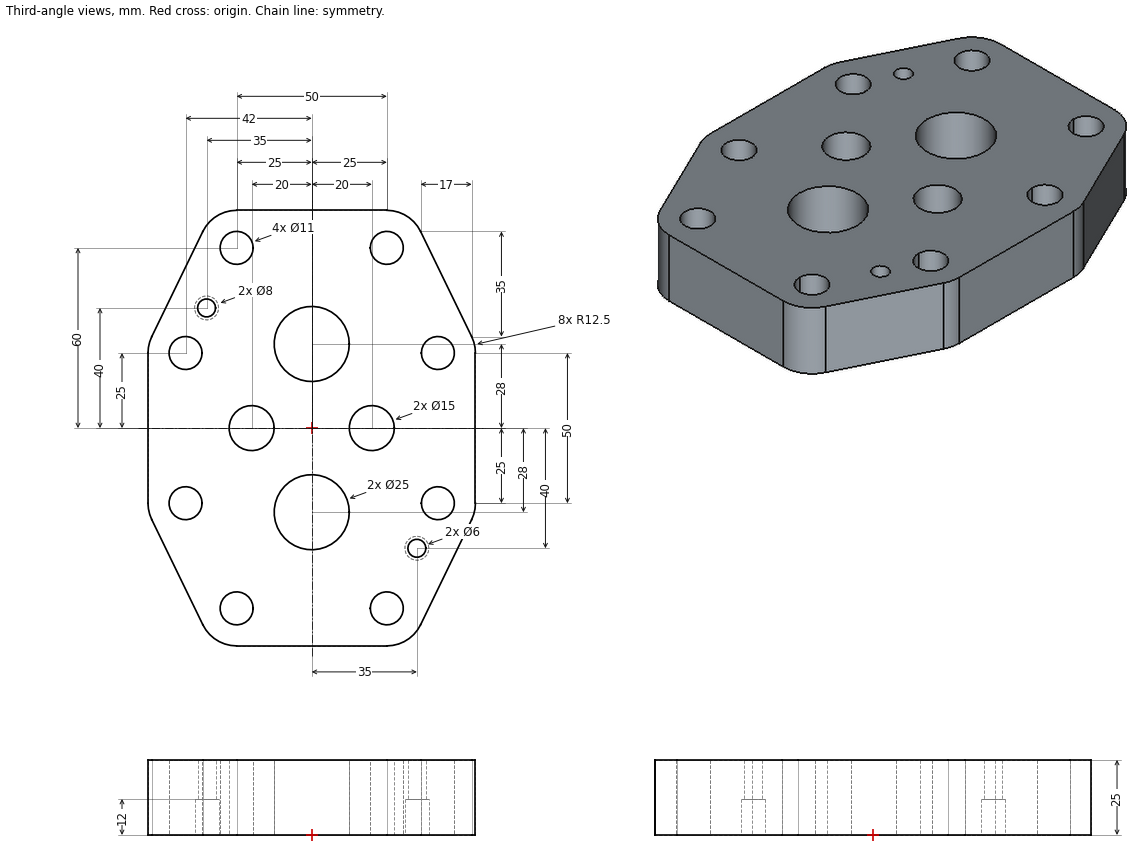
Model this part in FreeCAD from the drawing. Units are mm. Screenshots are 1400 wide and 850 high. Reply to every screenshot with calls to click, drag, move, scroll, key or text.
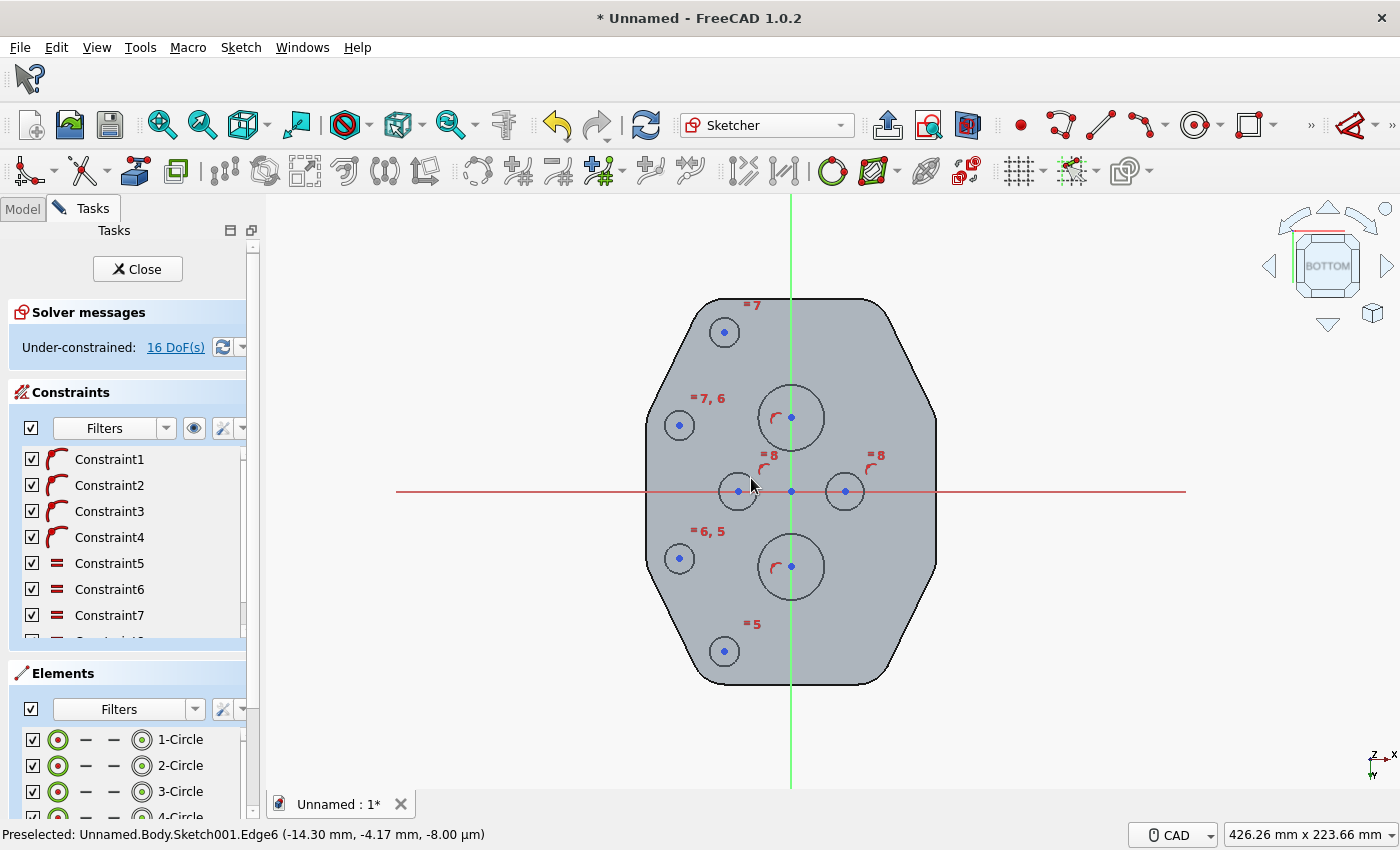
click(815, 395)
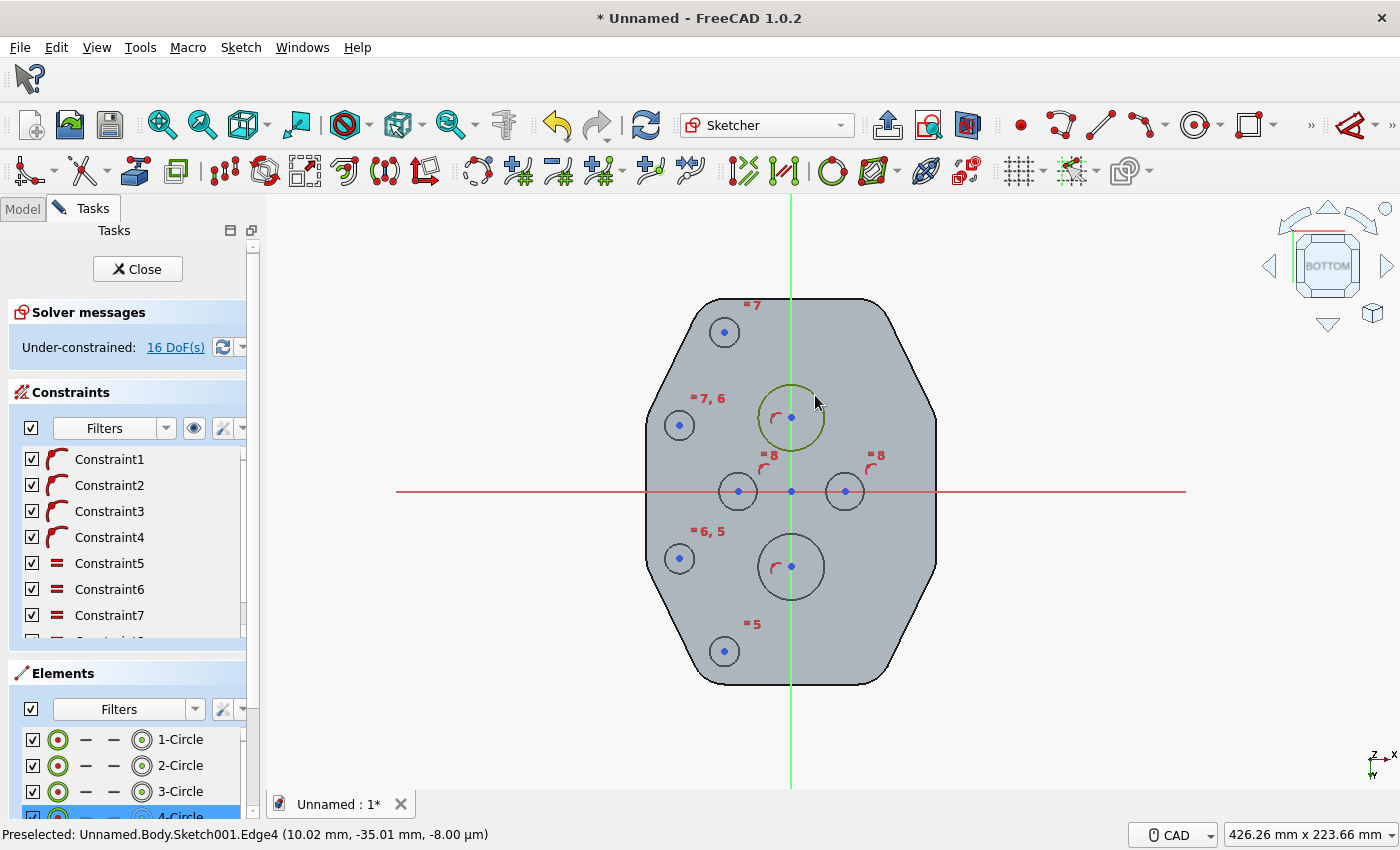
click(815, 544)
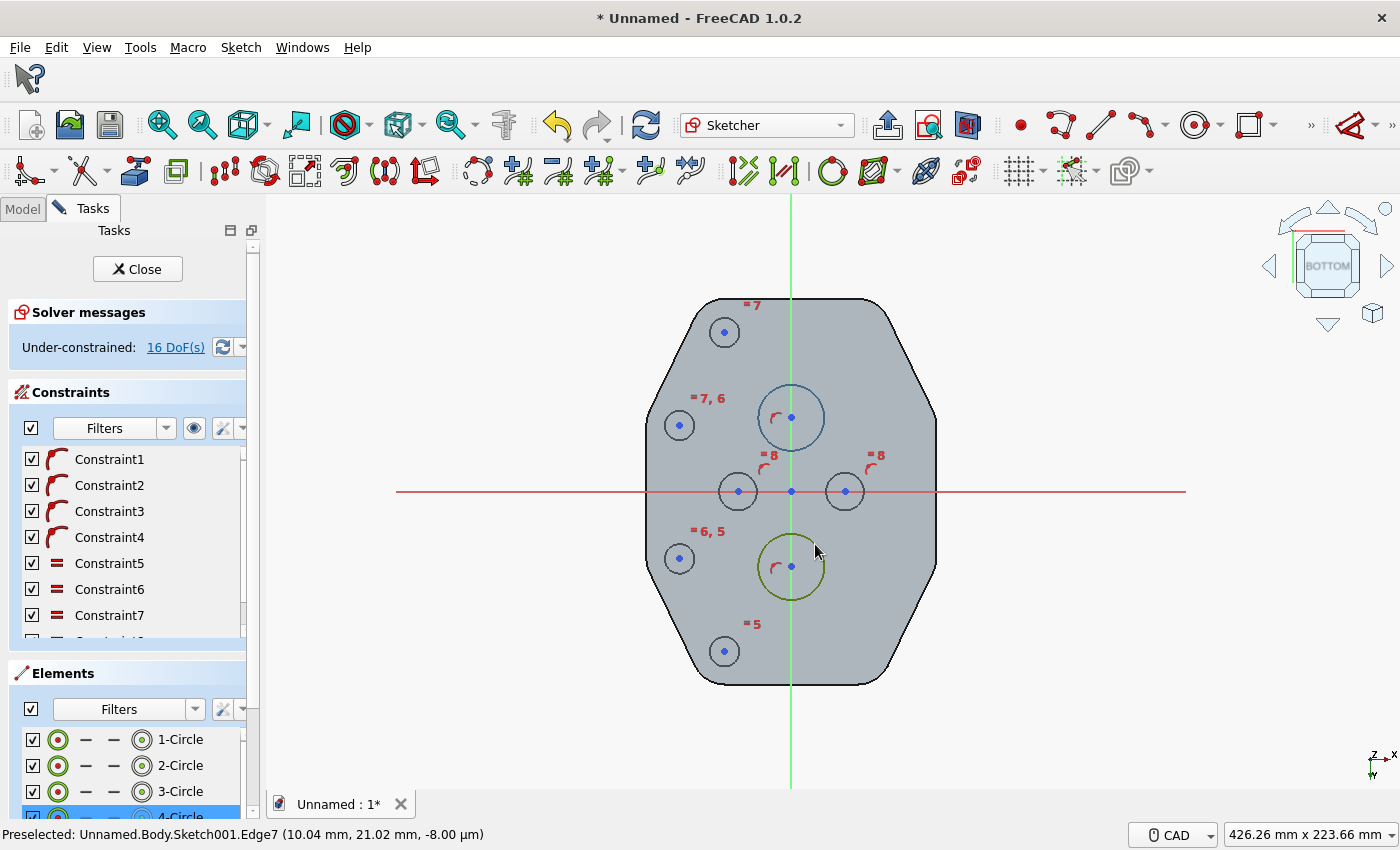
key(e)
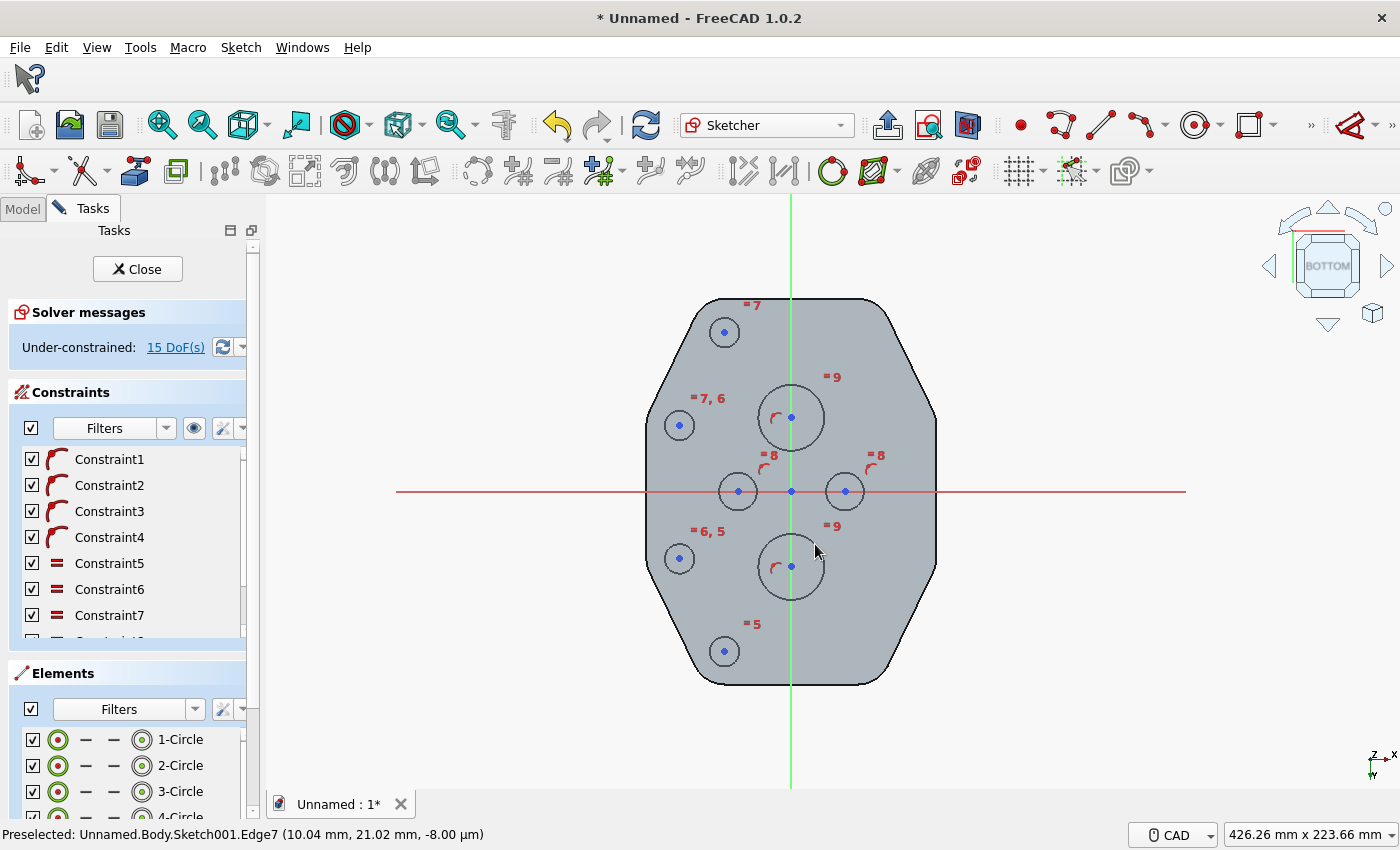
click(680, 559)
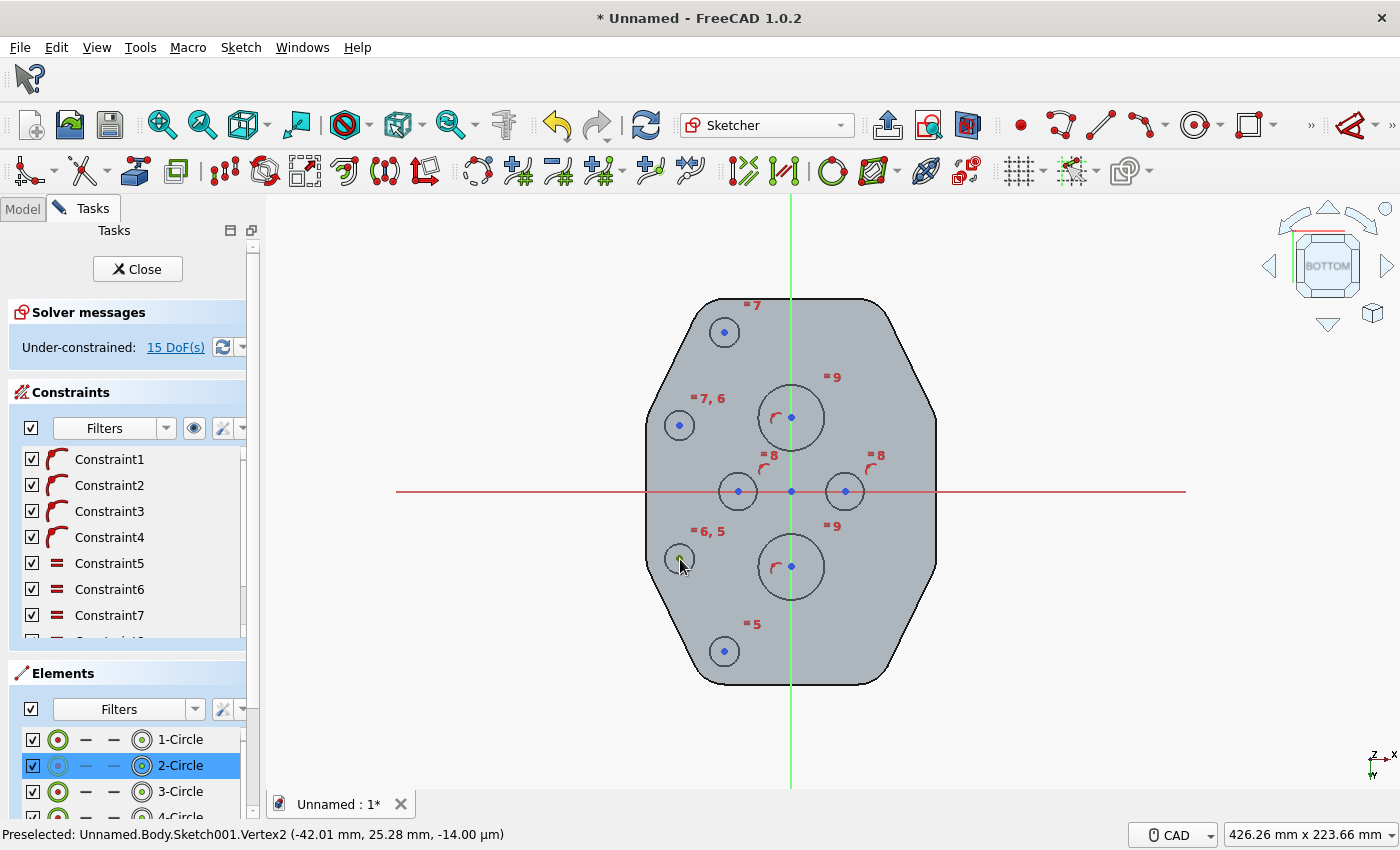
click(680, 426)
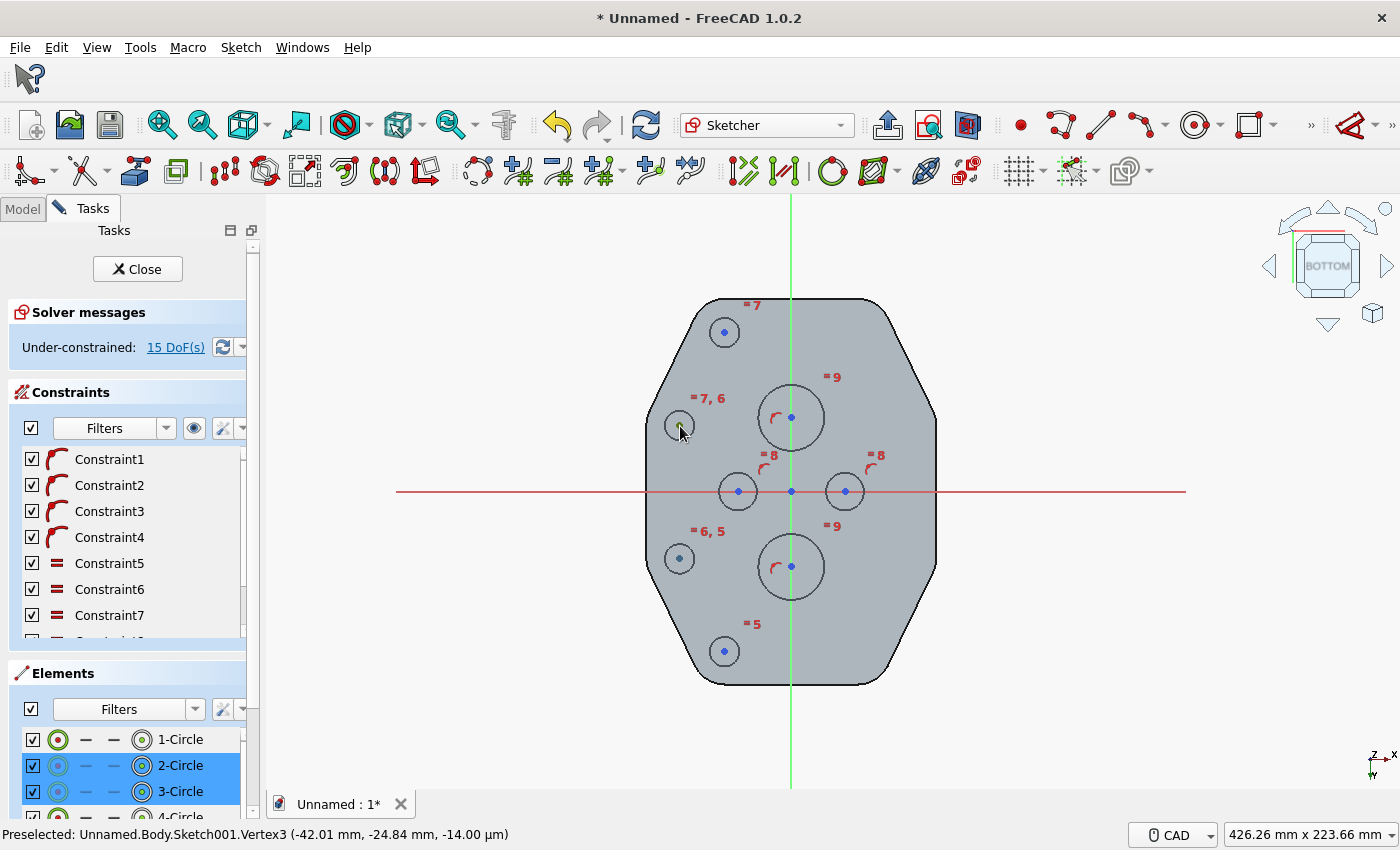
key(v)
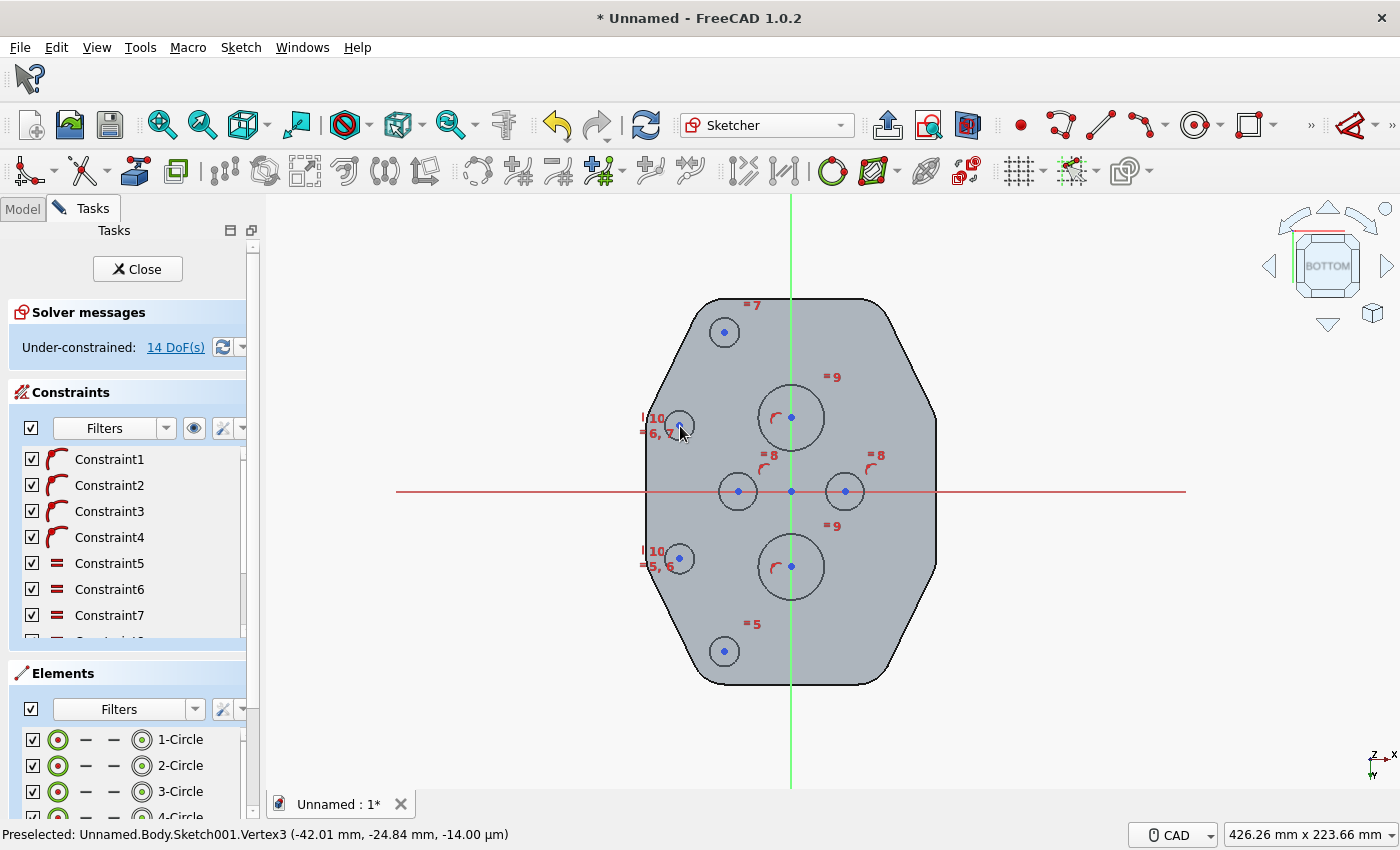
click(725, 652)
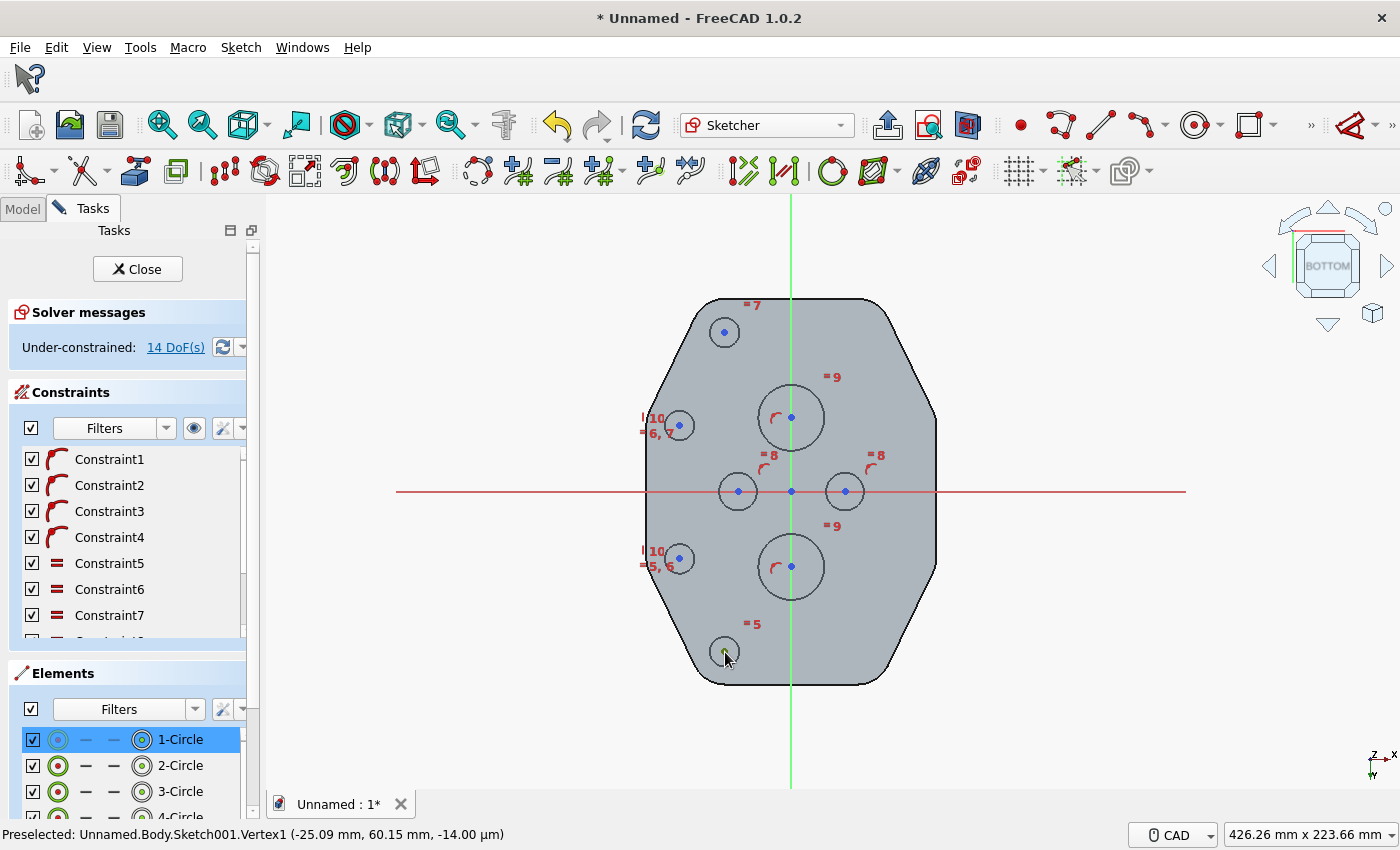
click(725, 333)